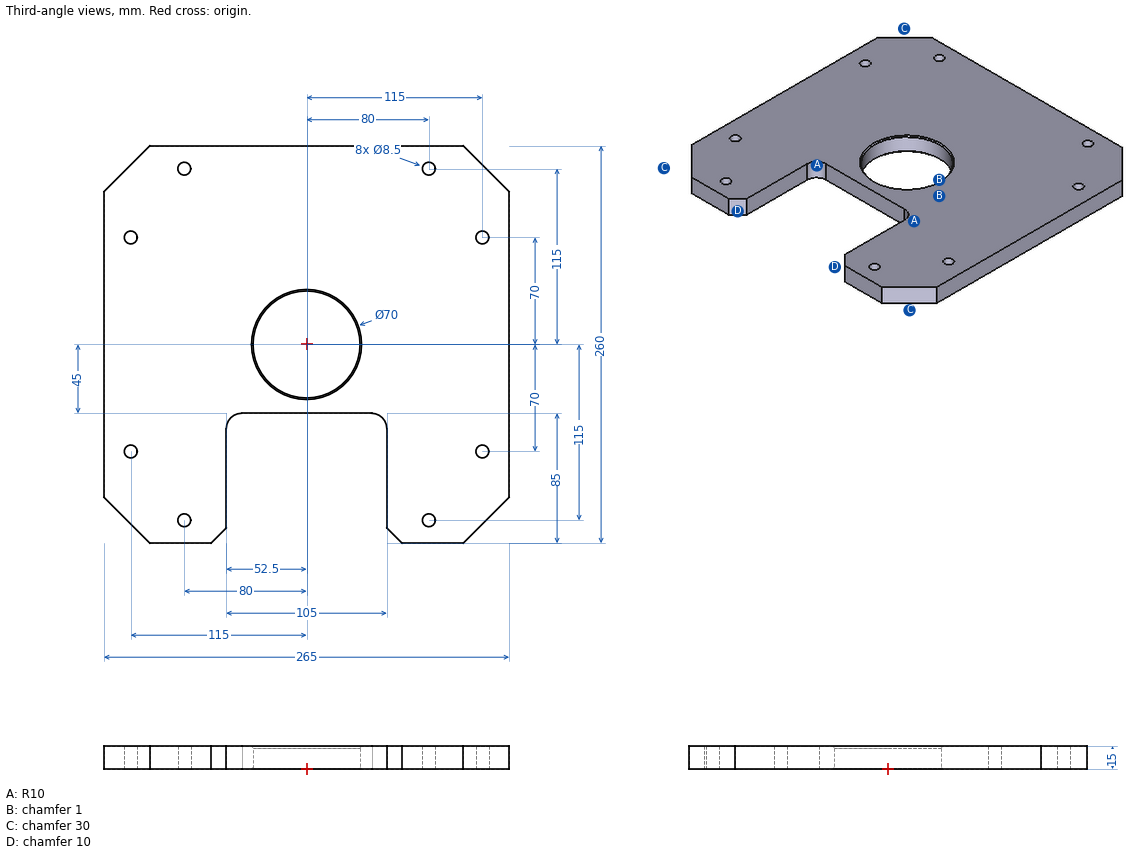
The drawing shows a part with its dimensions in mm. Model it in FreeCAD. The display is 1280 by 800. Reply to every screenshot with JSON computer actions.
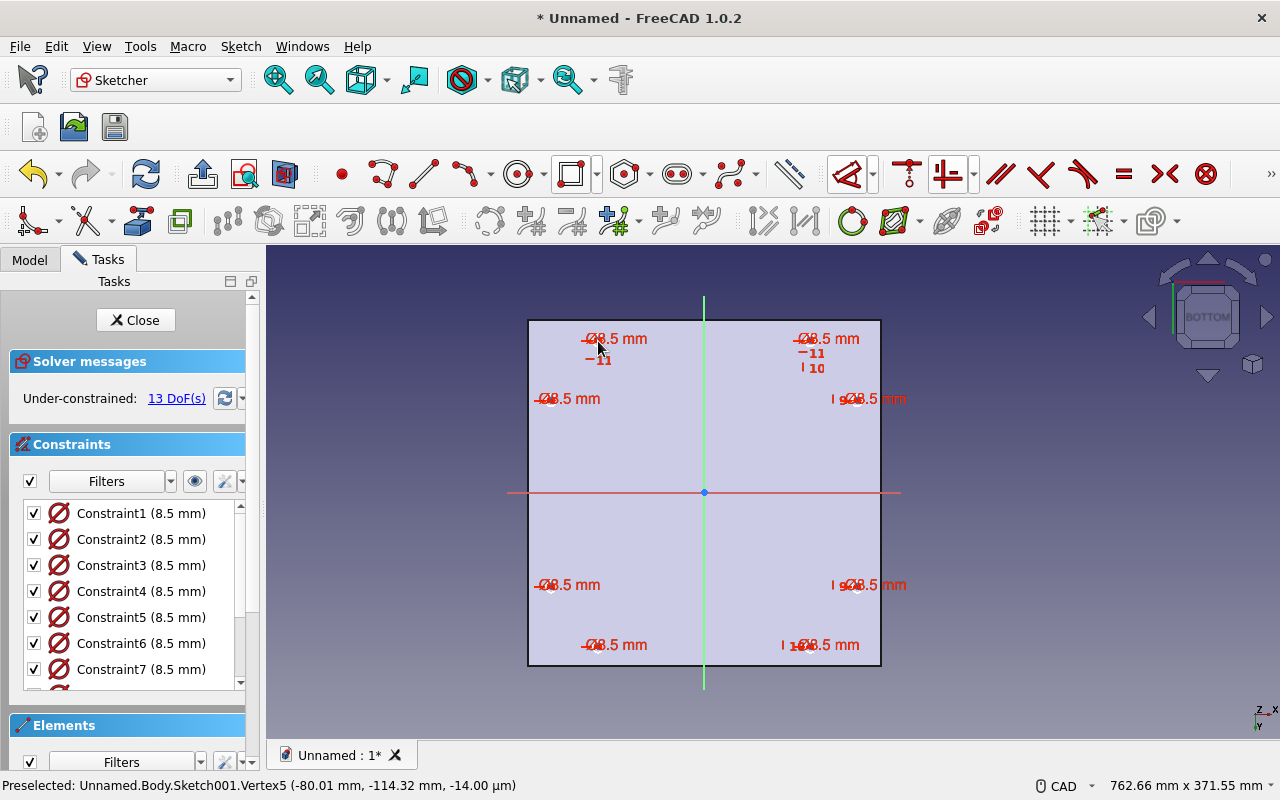
{"action": "left_click", "coordinate": [857, 401]}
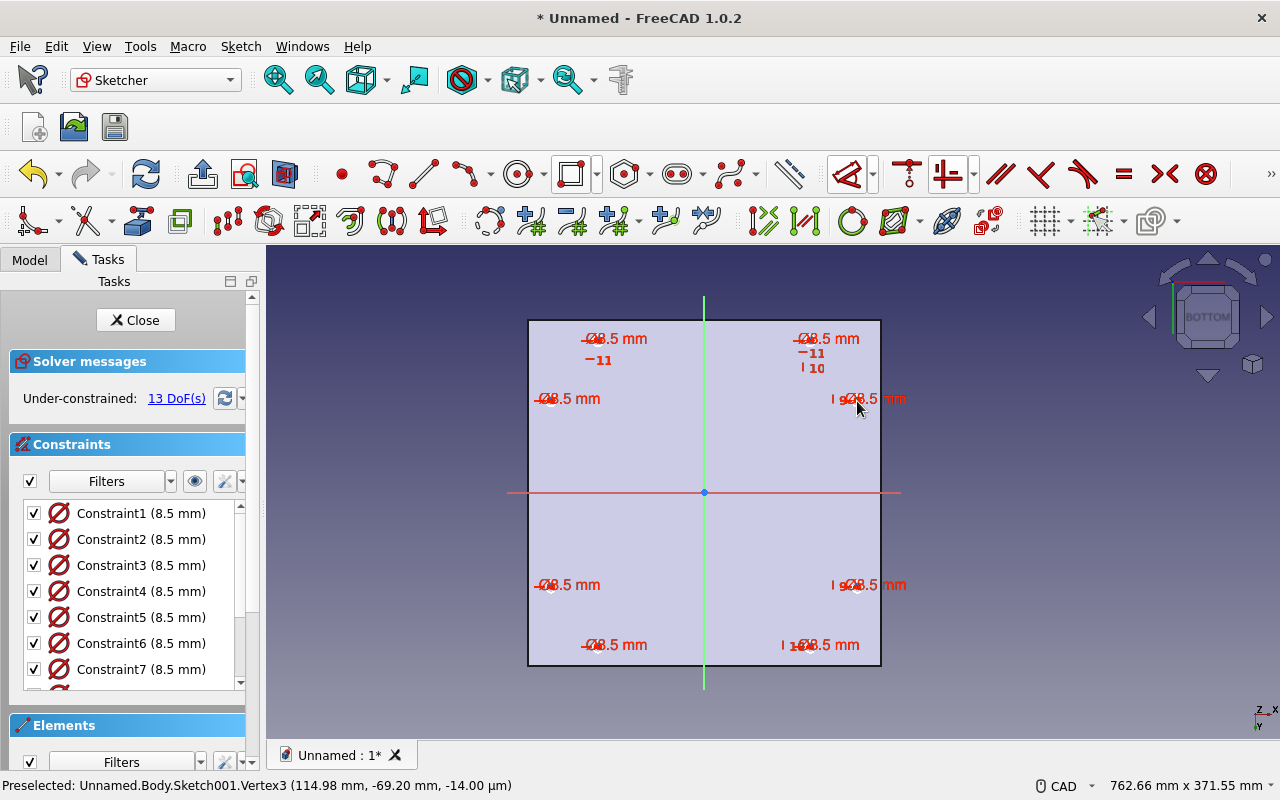
{"action": "left_click", "coordinate": [551, 401]}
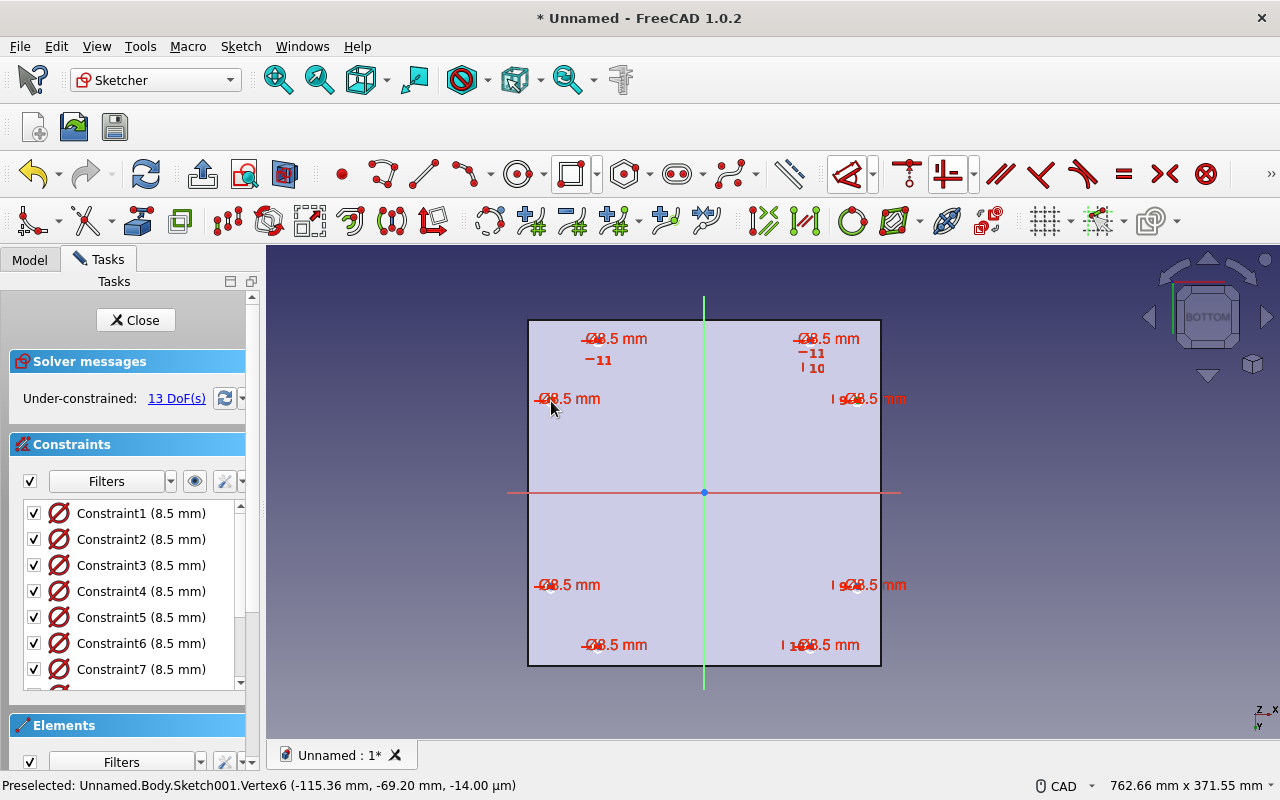
{"action": "left_click", "coordinate": [974, 174]}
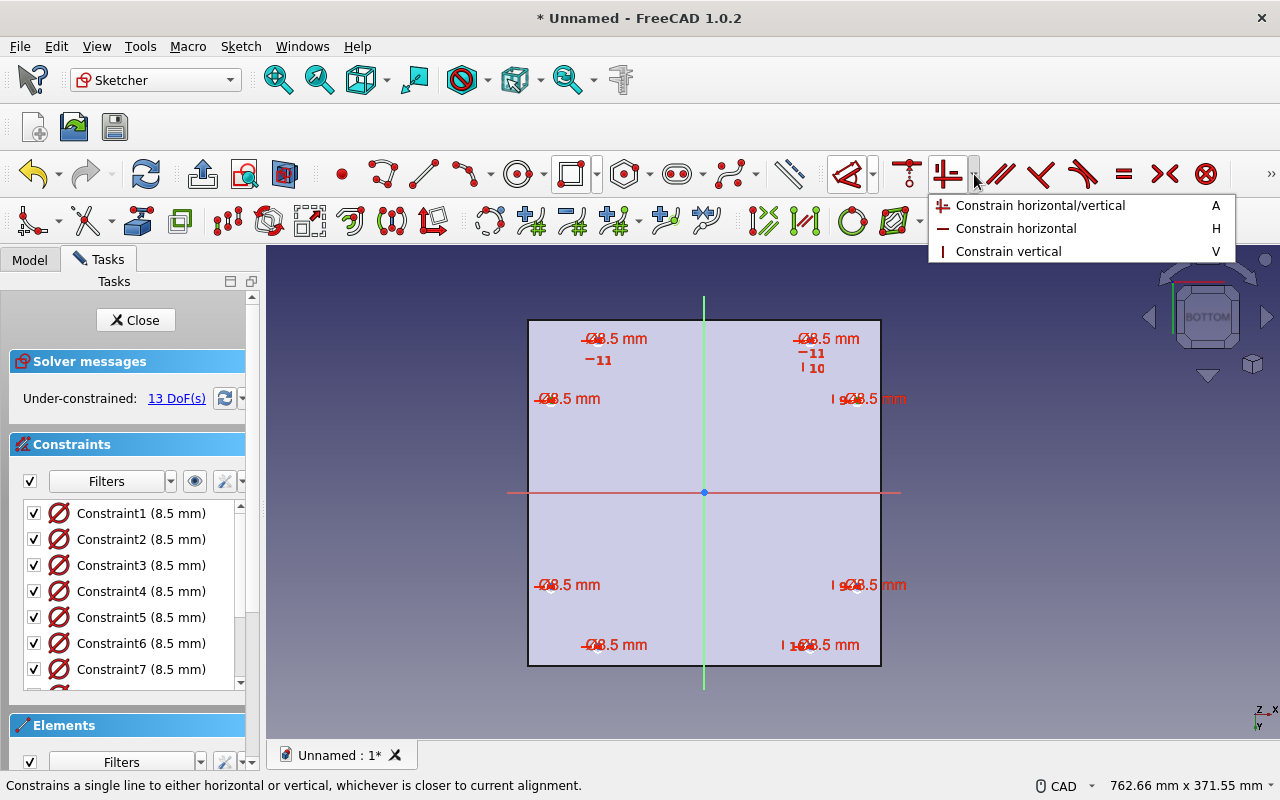
{"action": "left_click", "coordinate": [1082, 228]}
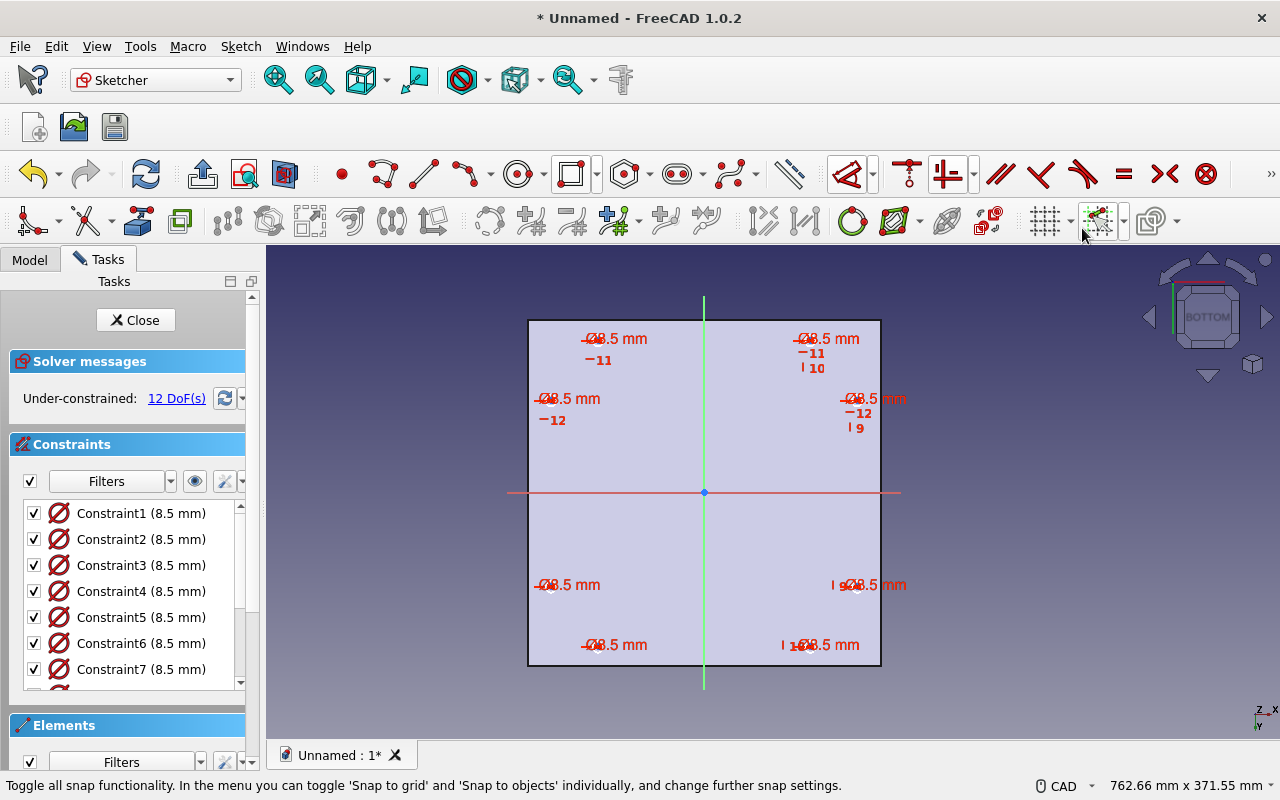
{"action": "left_click", "coordinate": [551, 401]}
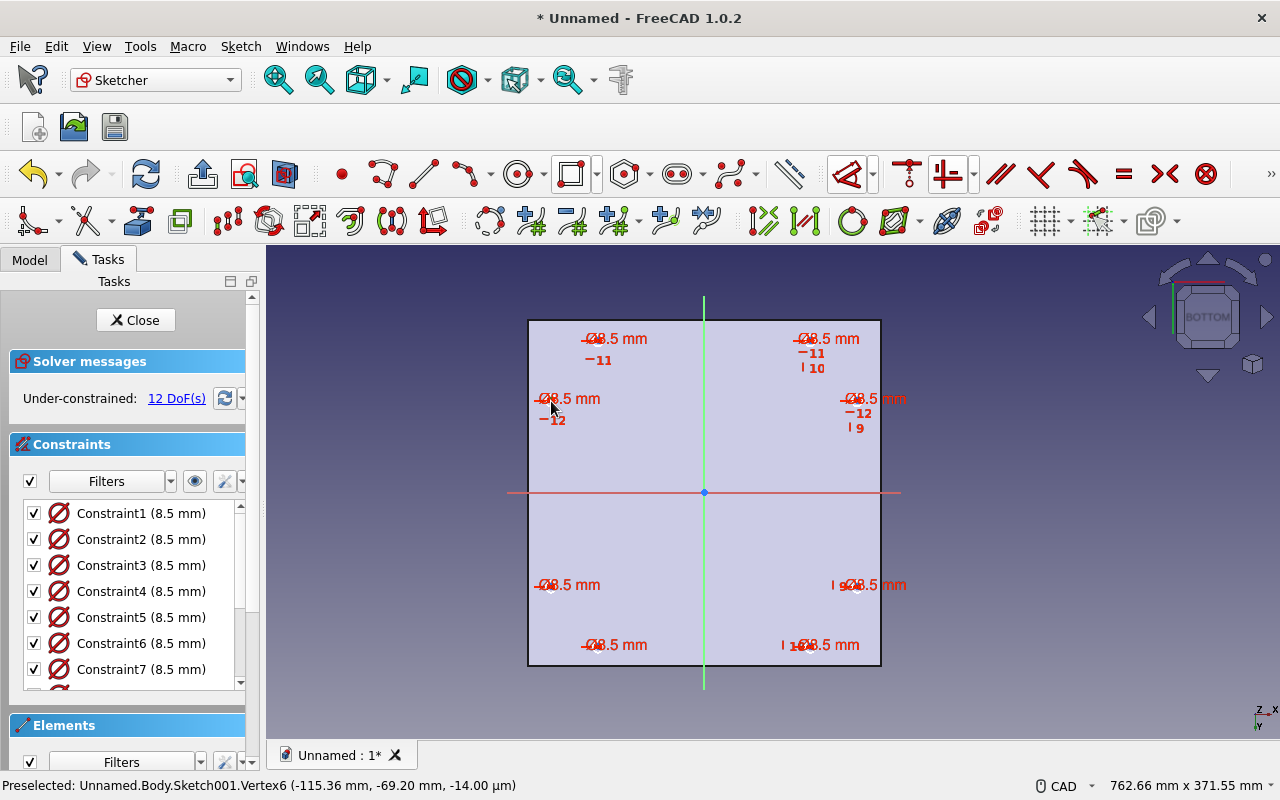
{"action": "left_click", "coordinate": [551, 587]}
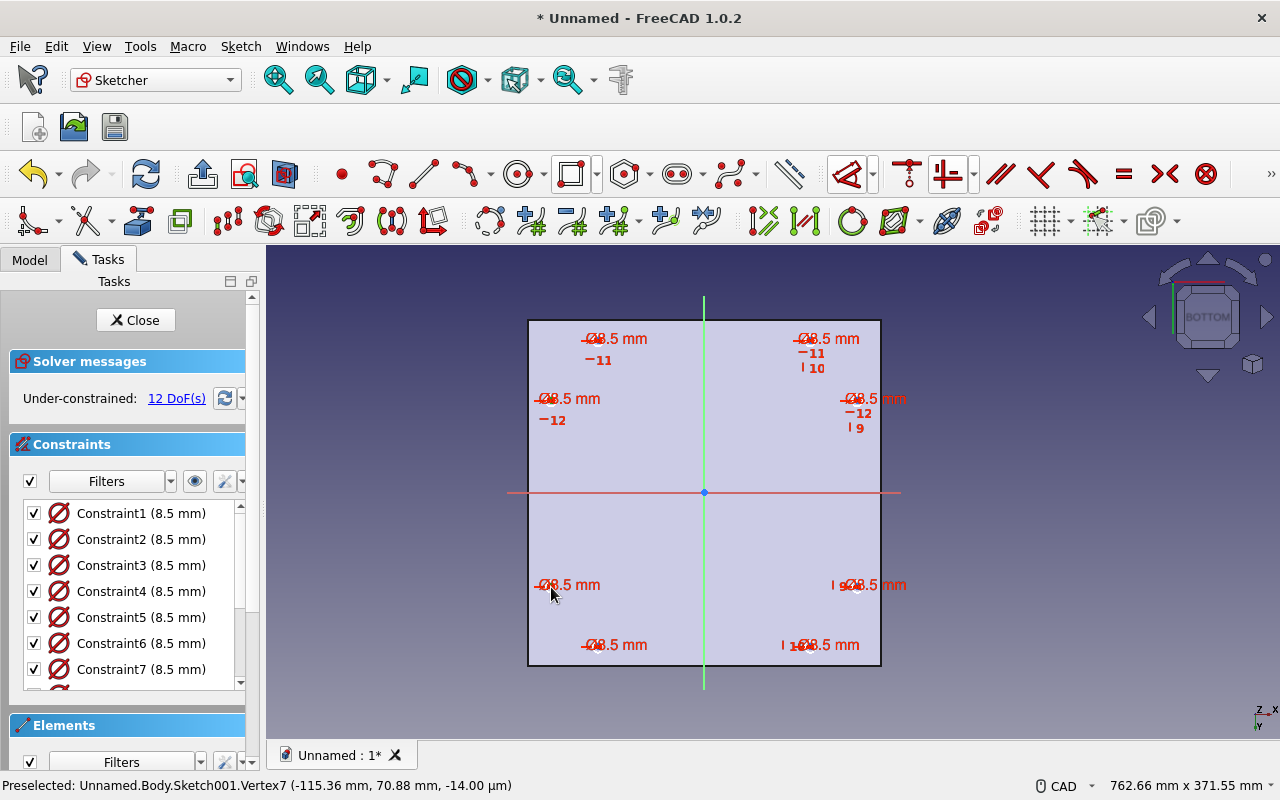
{"action": "key", "text": "v"}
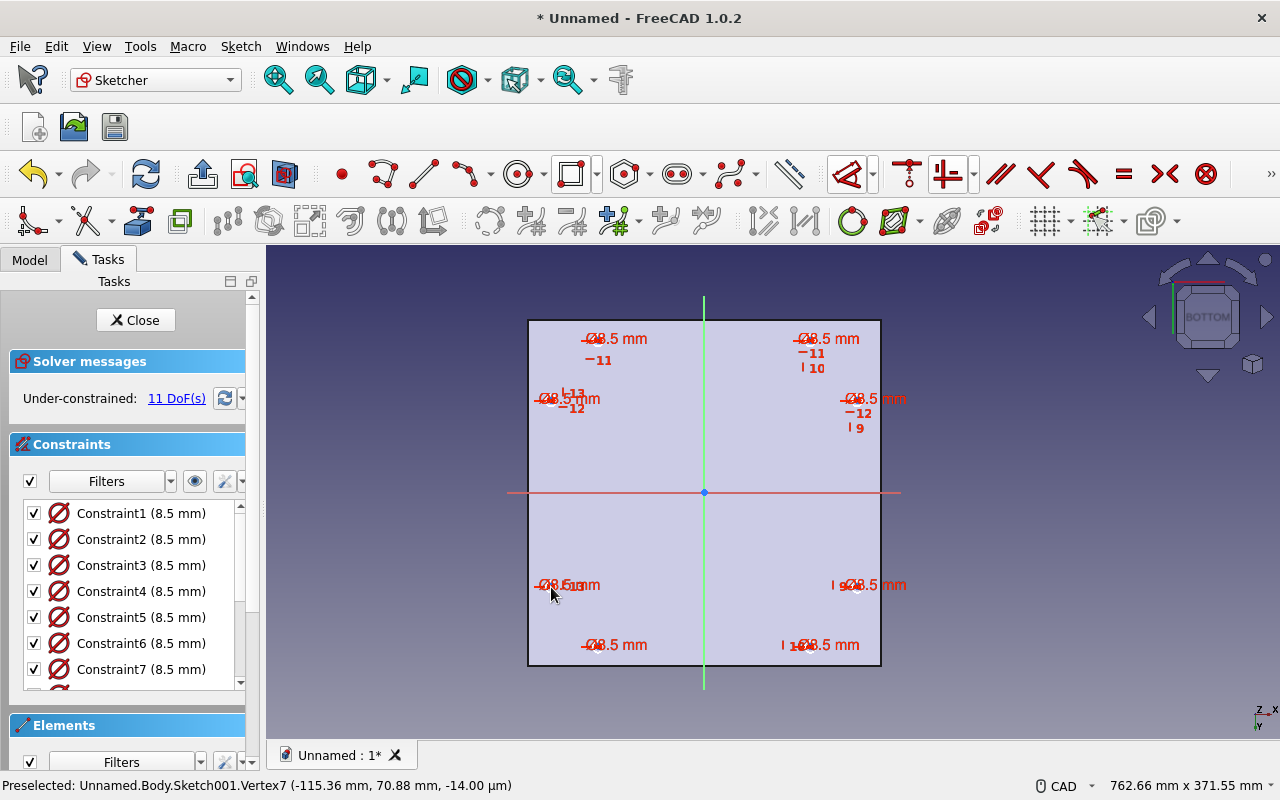
{"action": "left_click", "coordinate": [857, 587]}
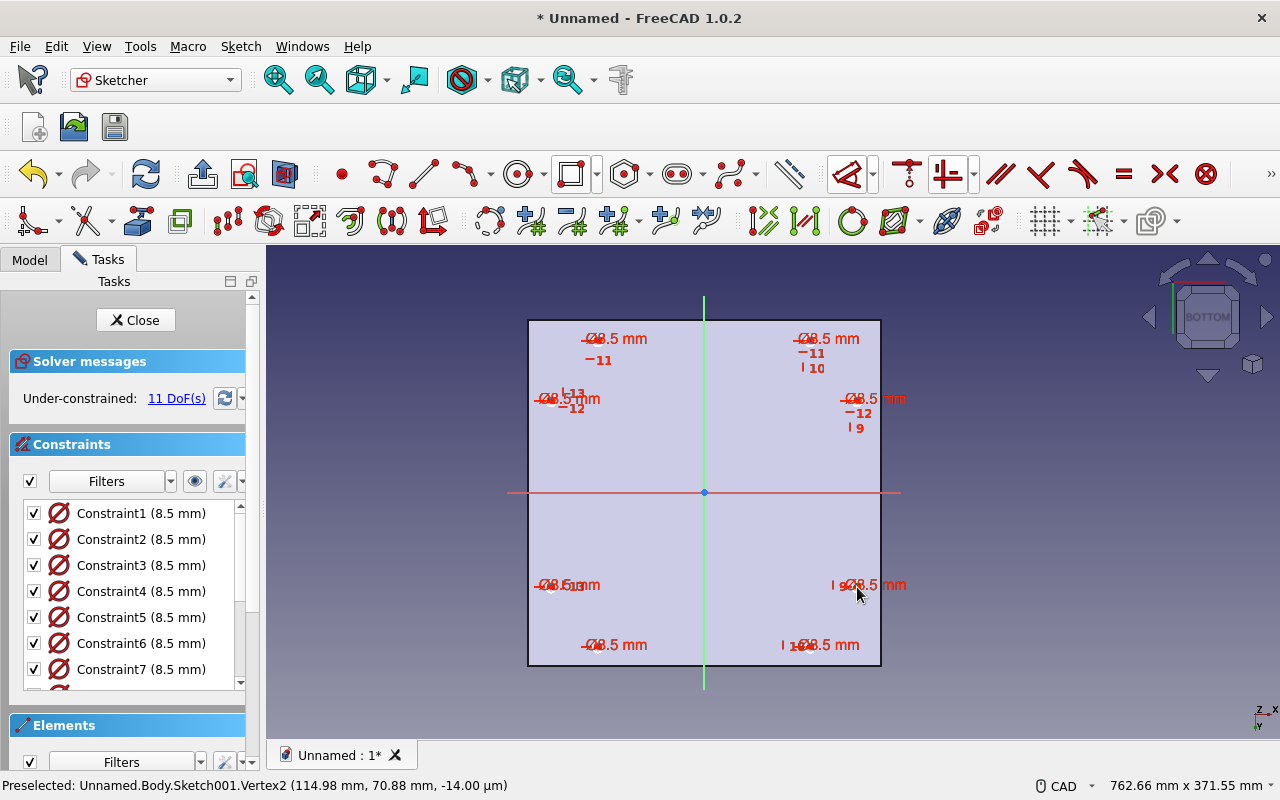
{"action": "left_click", "coordinate": [551, 587]}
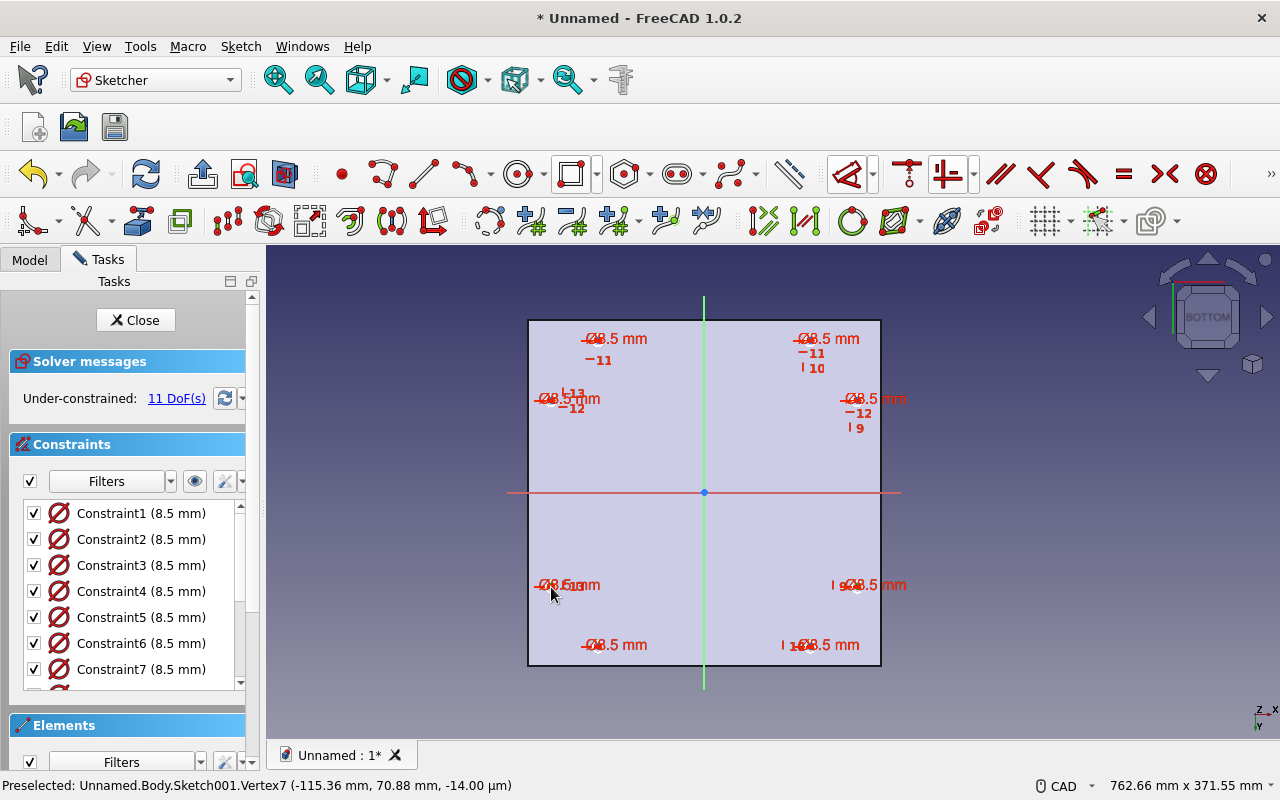
{"action": "key", "text": "h"}